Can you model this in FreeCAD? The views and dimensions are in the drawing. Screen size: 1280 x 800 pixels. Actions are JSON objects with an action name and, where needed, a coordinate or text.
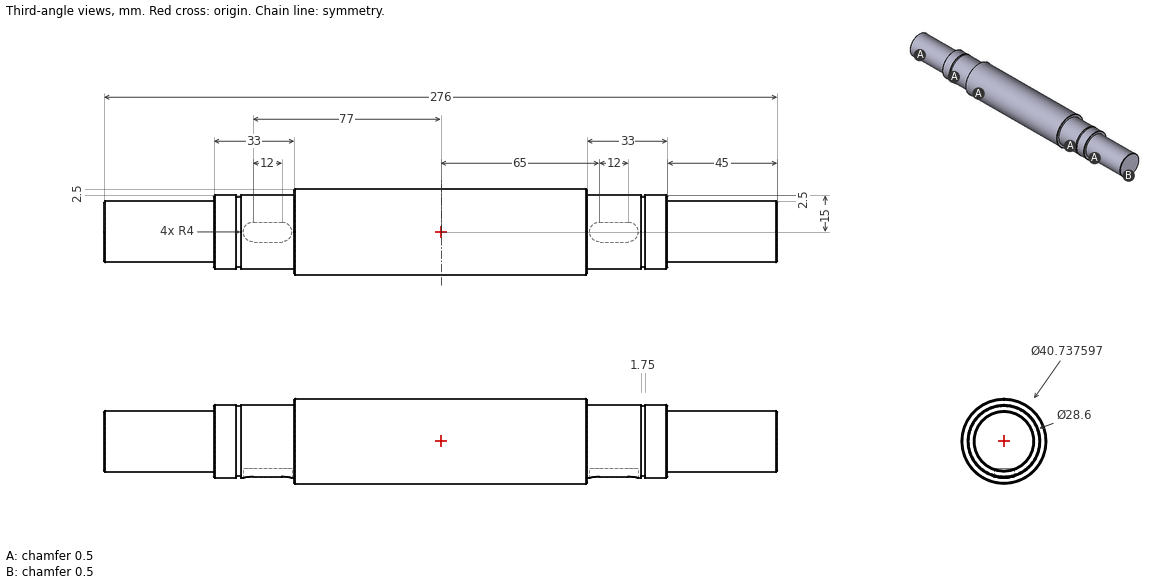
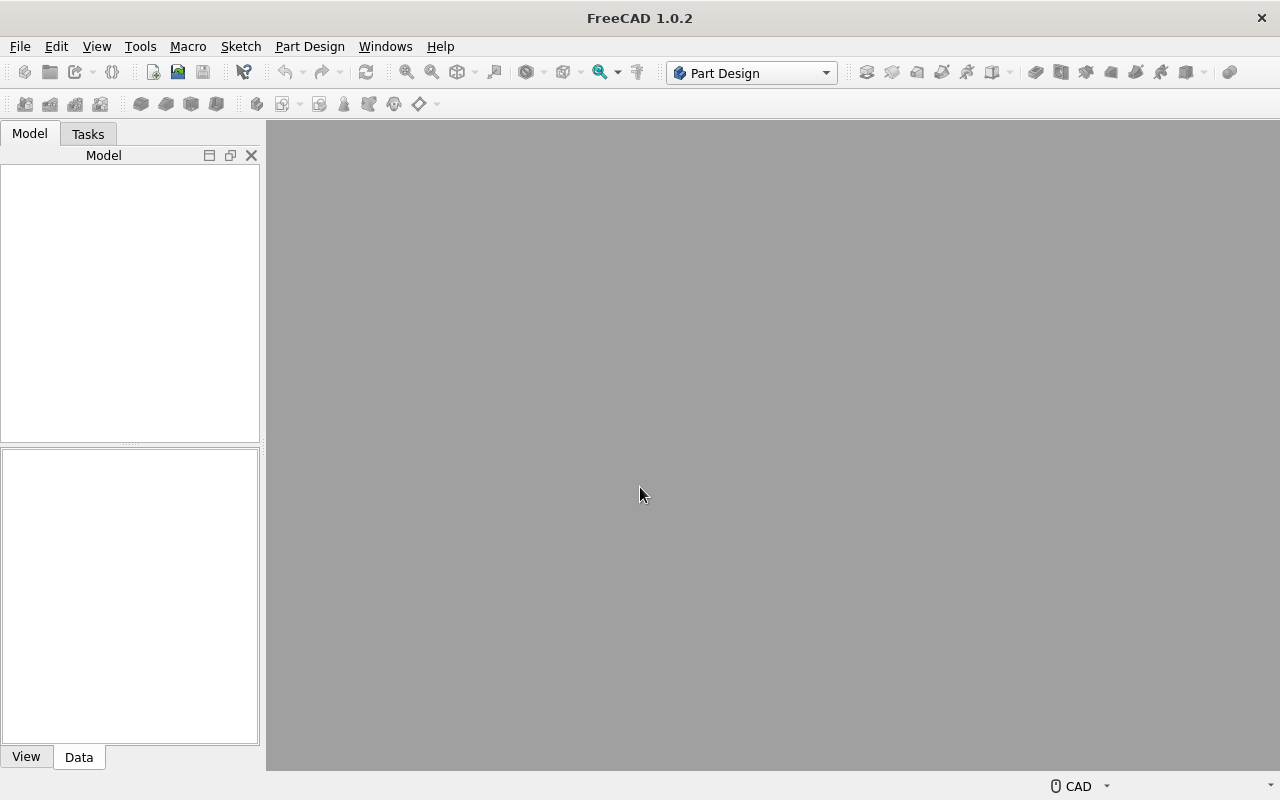
{"action": "left_click", "coordinate": [153, 72]}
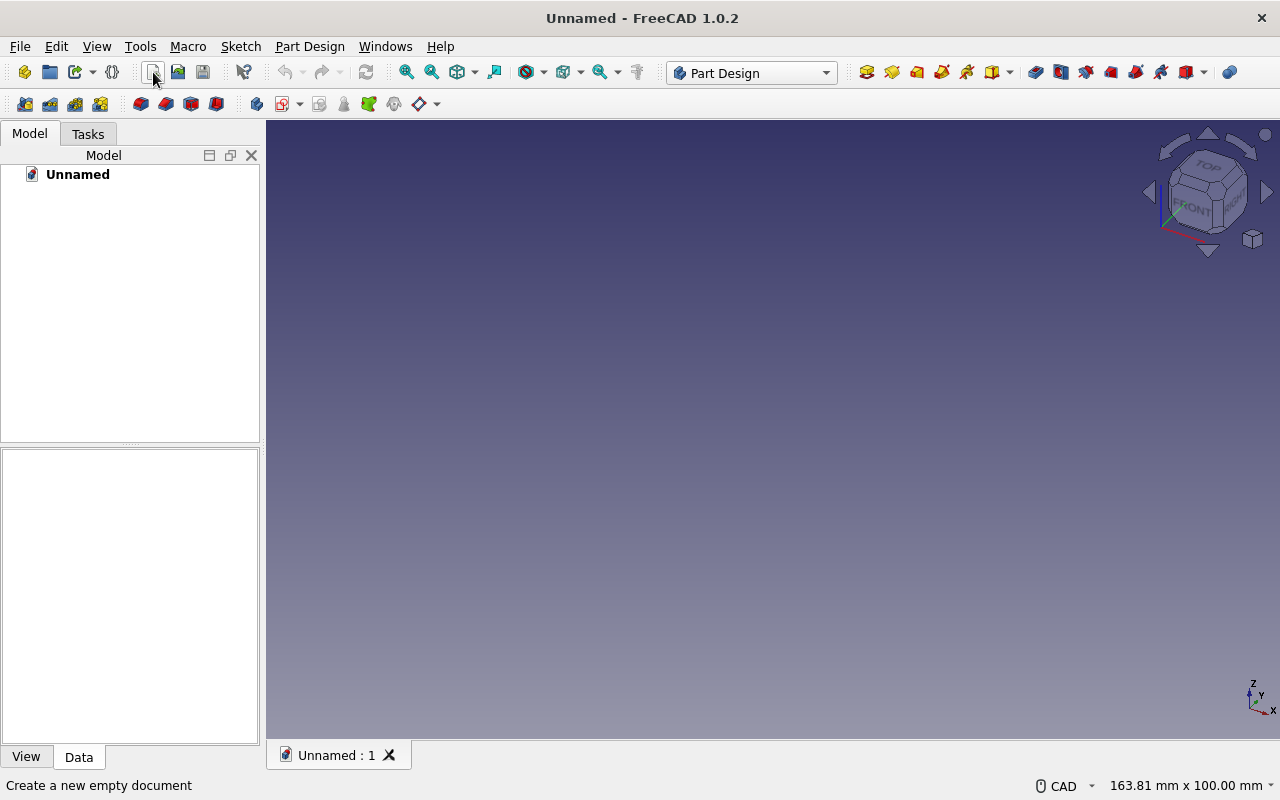
{"action": "left_click", "coordinate": [282, 104]}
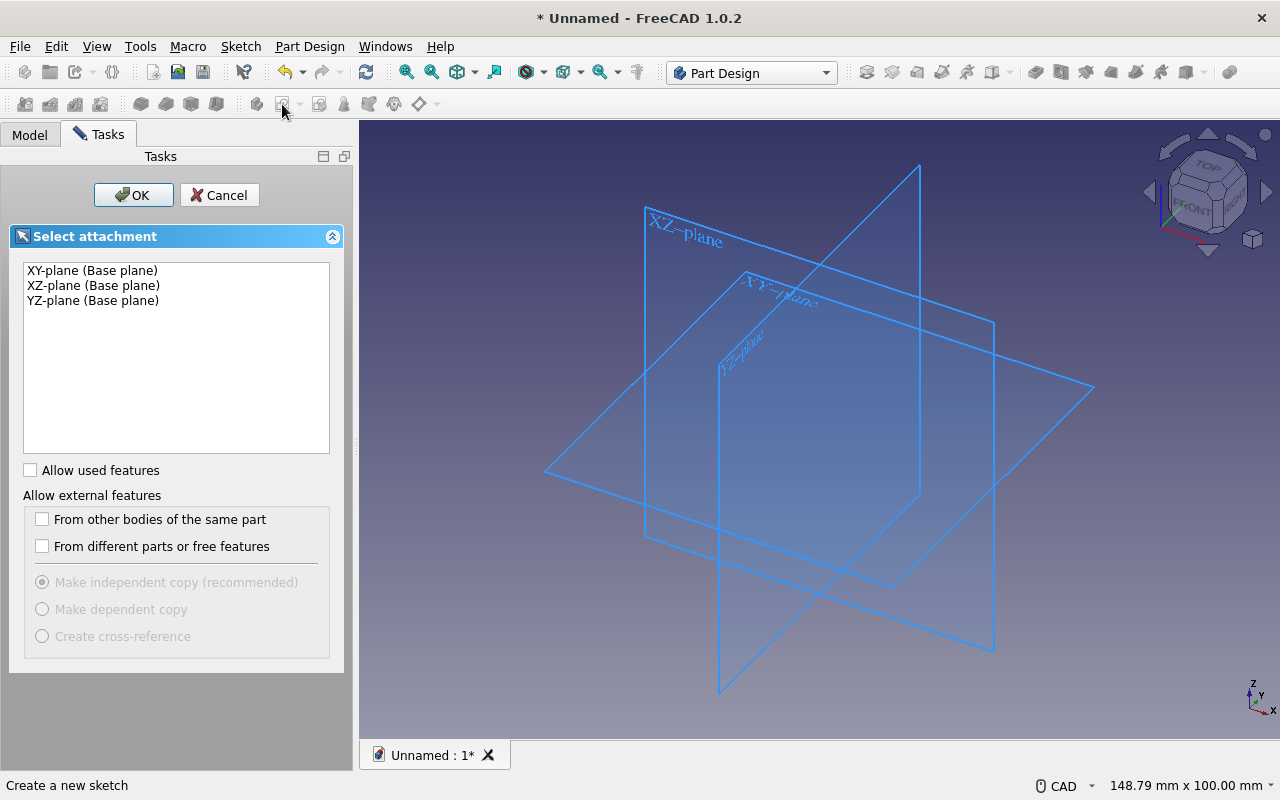
{"action": "left_click", "coordinate": [84, 270]}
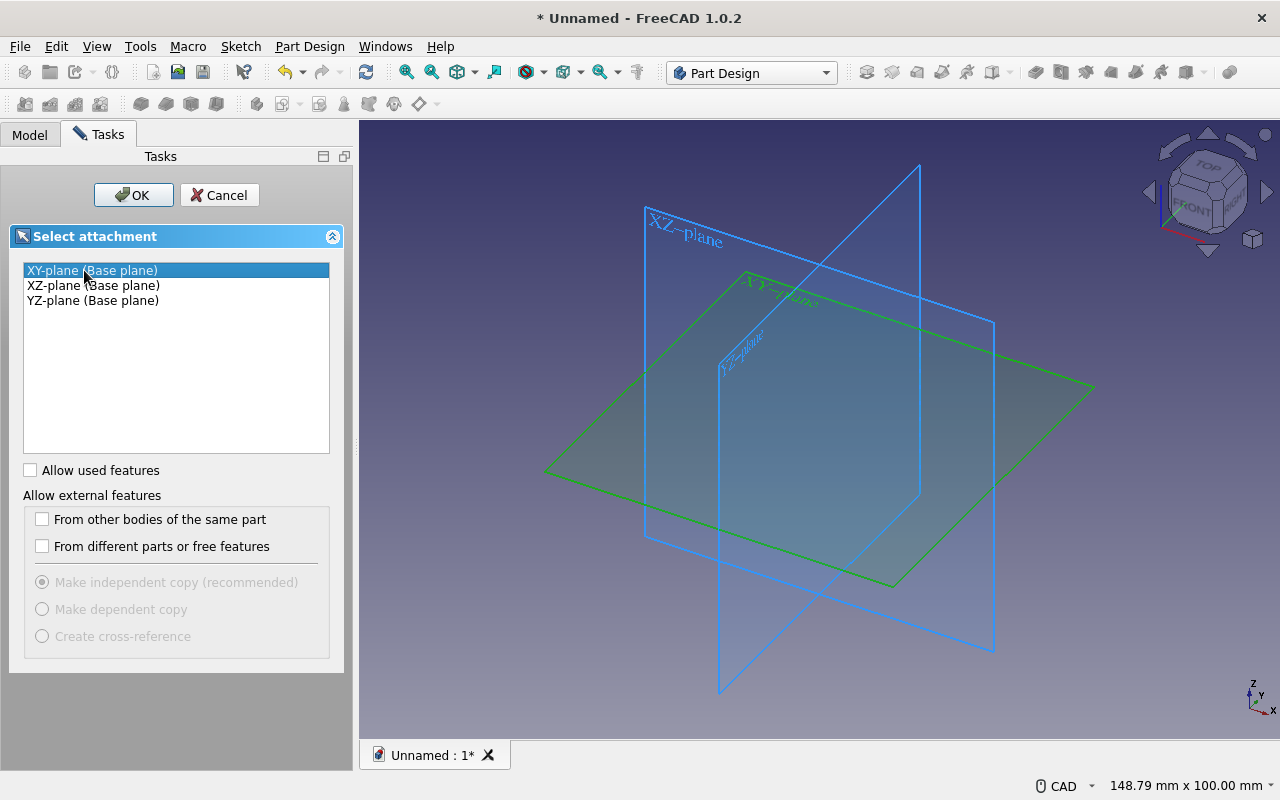
{"action": "left_click", "coordinate": [134, 195]}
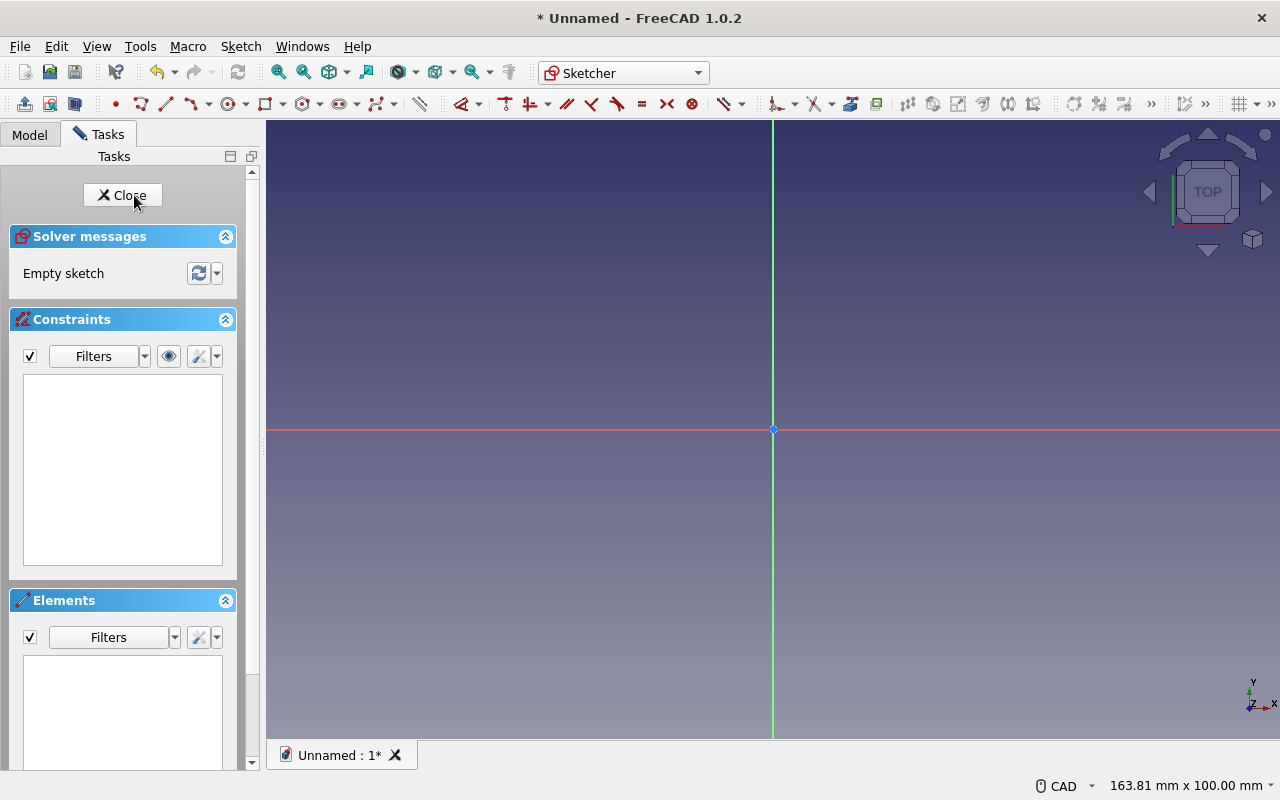
{"action": "scroll", "coordinate": [665, 461], "scroll_direction": "down", "scroll_amount": 5}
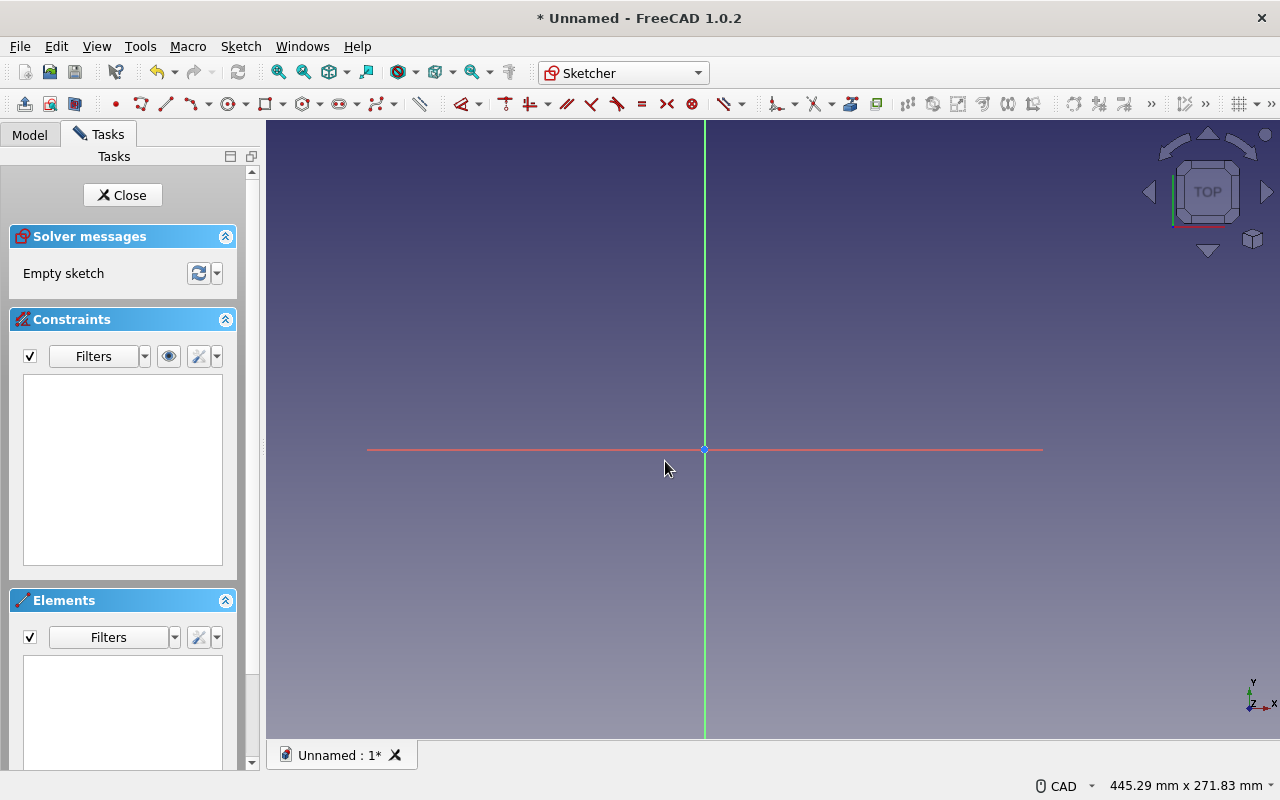
{"action": "left_click", "coordinate": [141, 104]}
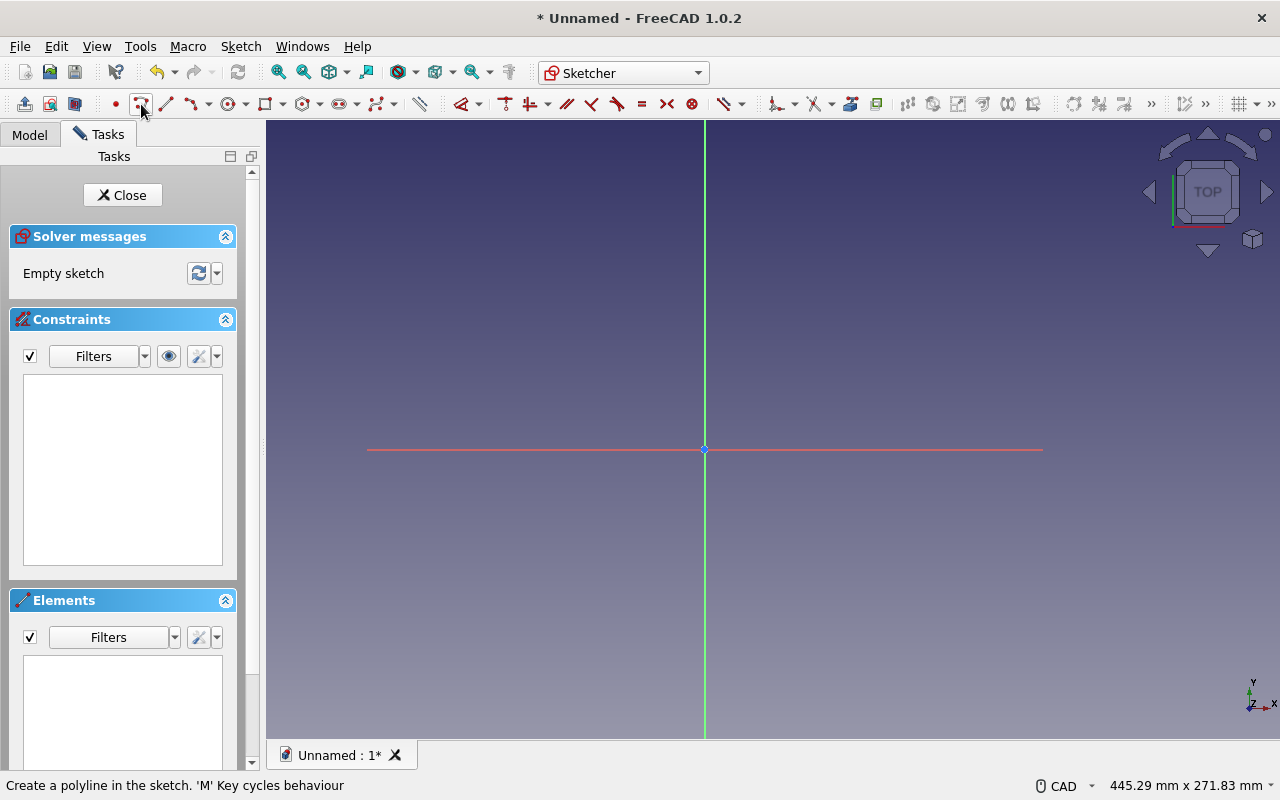
{"action": "left_click", "coordinate": [842, 416]}
{"action": "left_click", "coordinate": [917, 416]}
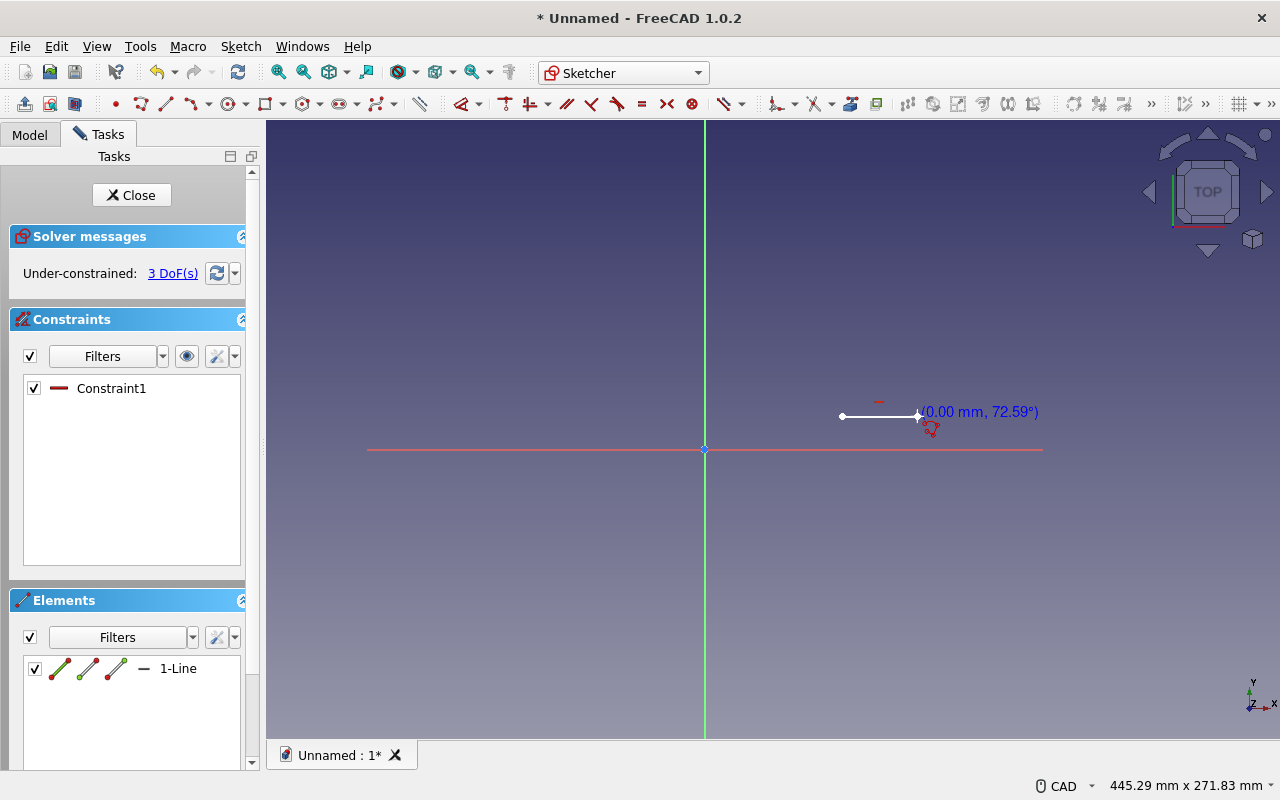
{"action": "scroll", "coordinate": [917, 421], "scroll_direction": "up", "scroll_amount": 6}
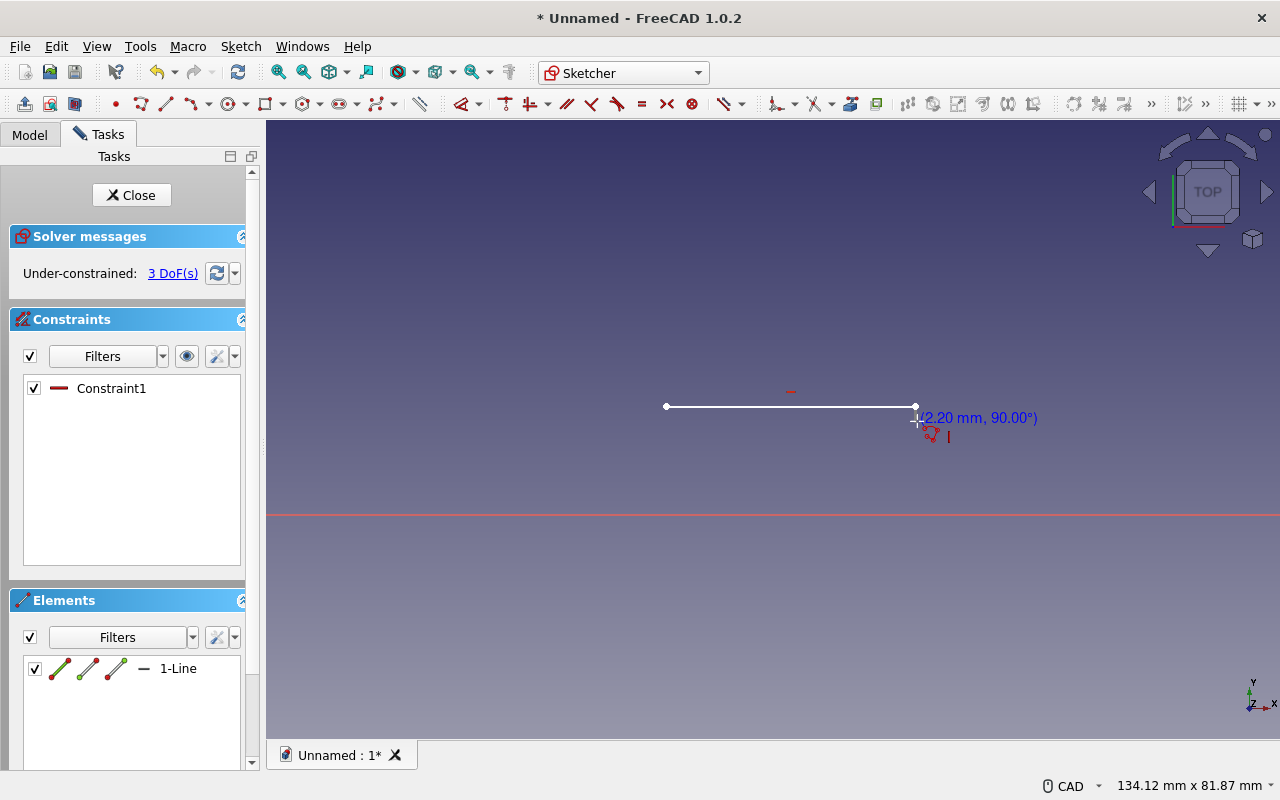
{"action": "left_click", "coordinate": [916, 421]}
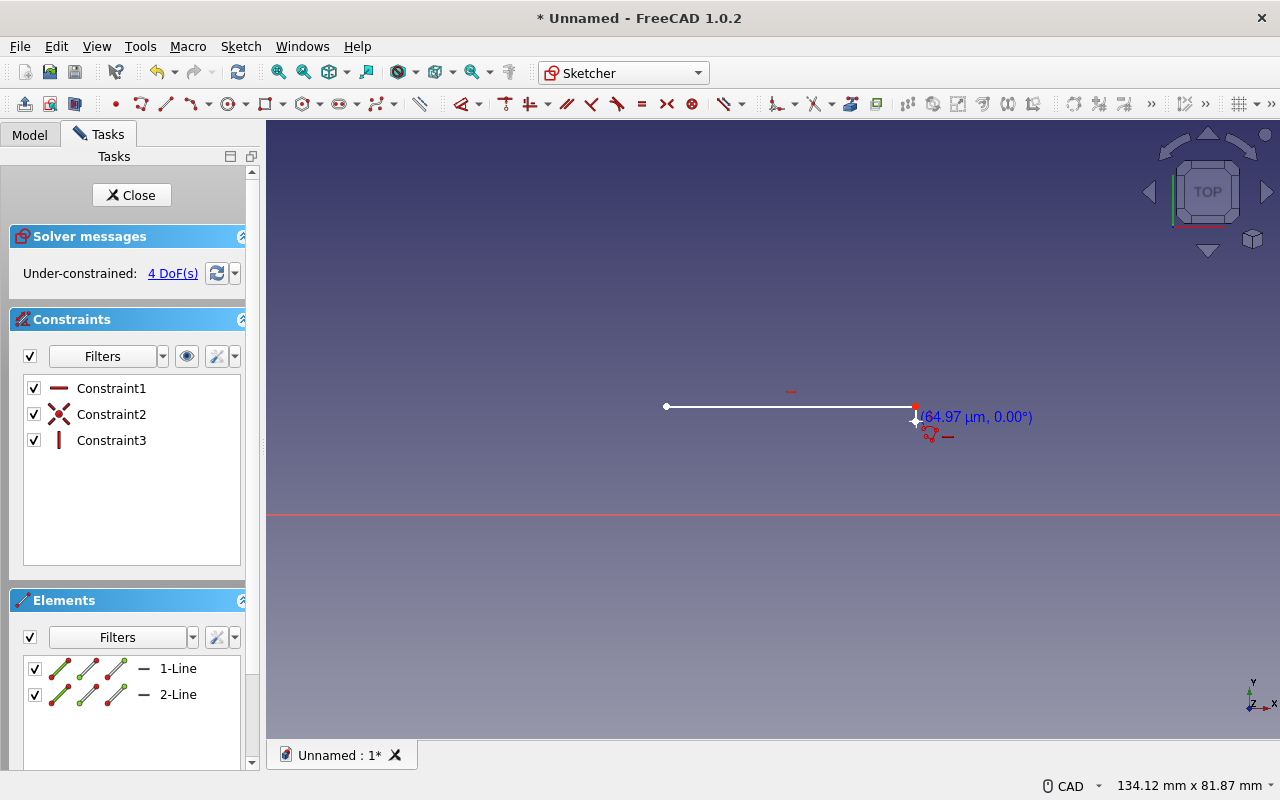
{"action": "scroll", "coordinate": [917, 421], "scroll_direction": "down", "scroll_amount": 6}